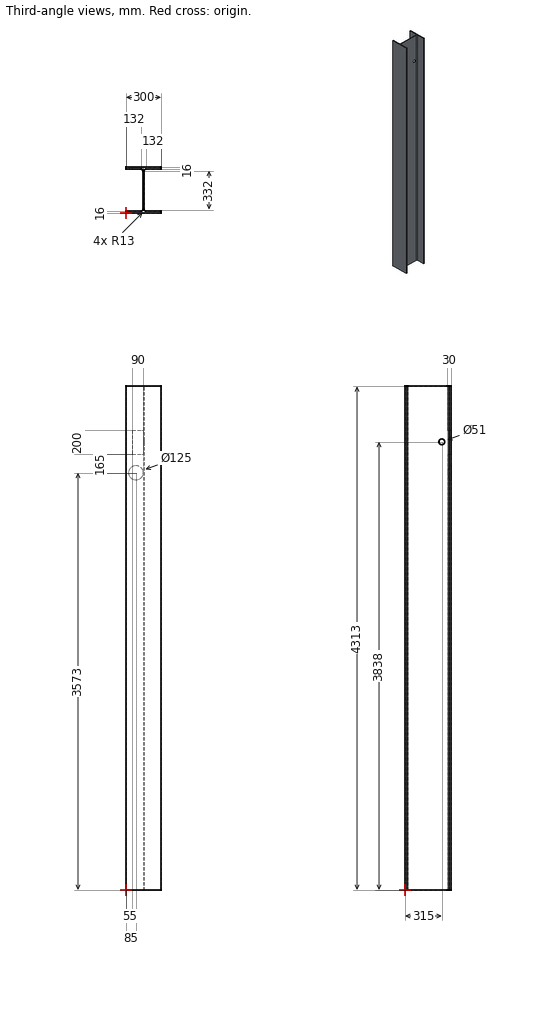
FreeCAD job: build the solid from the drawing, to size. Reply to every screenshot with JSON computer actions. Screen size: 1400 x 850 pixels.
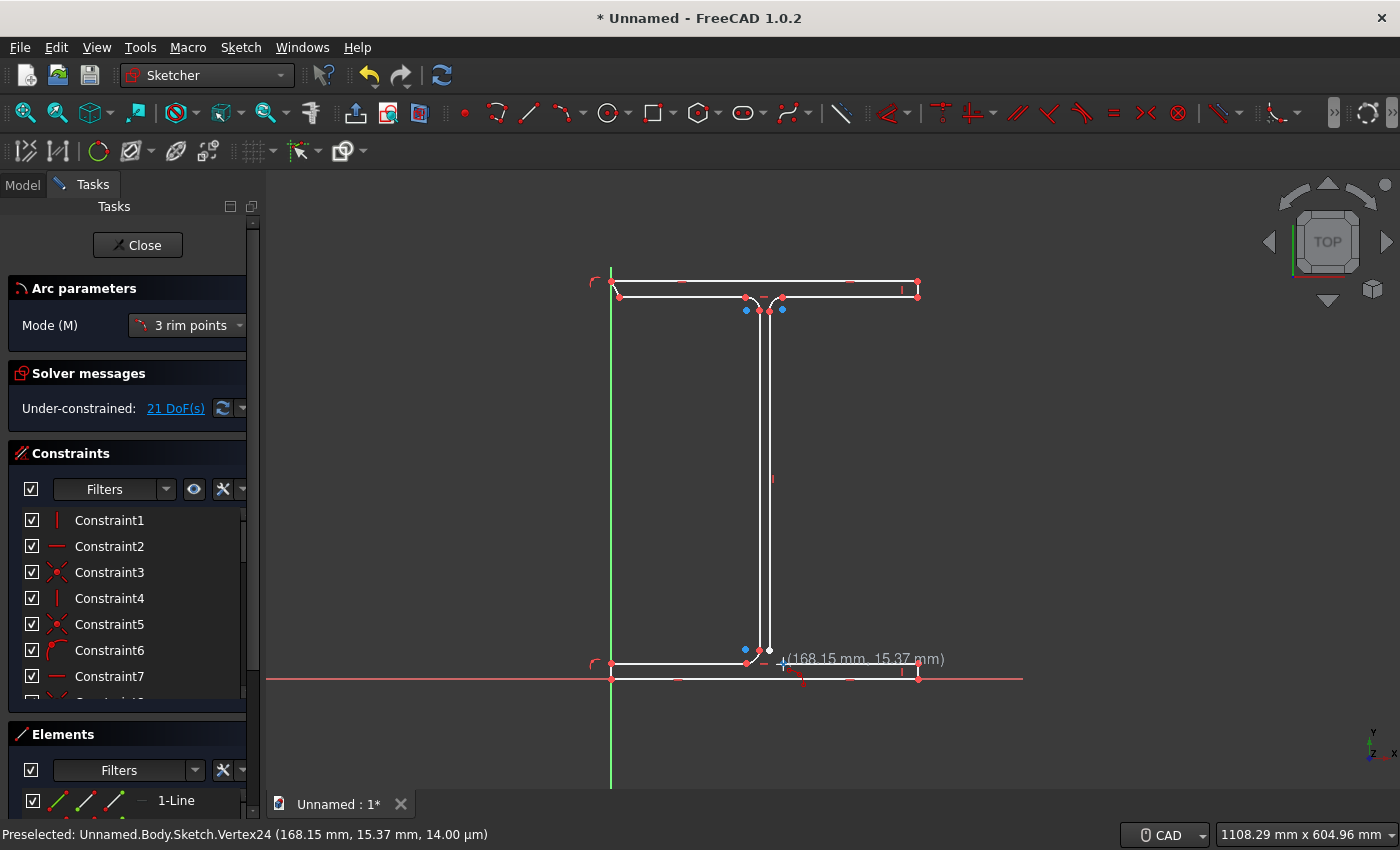
{"action": "scroll", "coordinate": [770, 650], "scroll_direction": "up", "scroll_amount": 3}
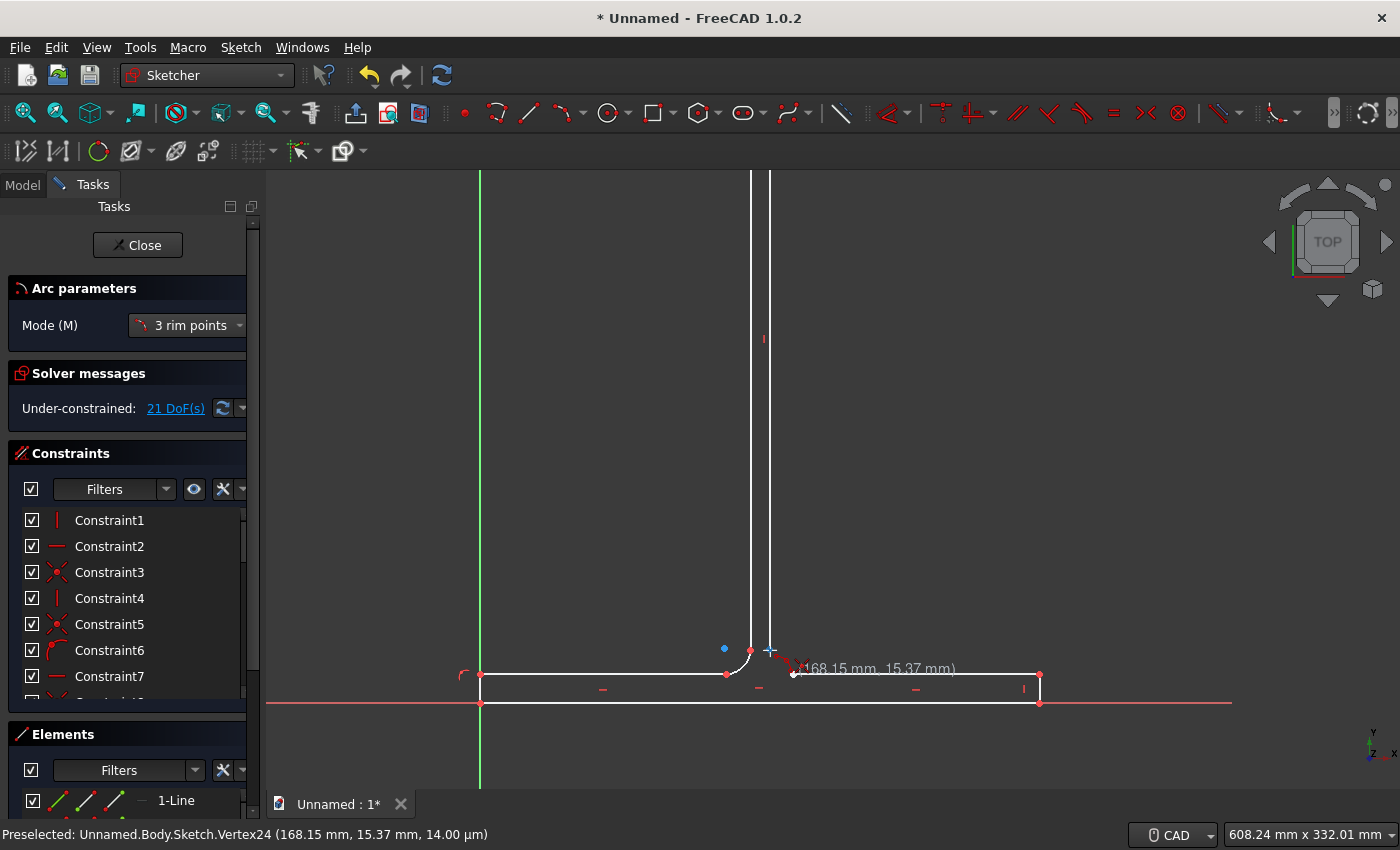
{"action": "left_click", "coordinate": [770, 650]}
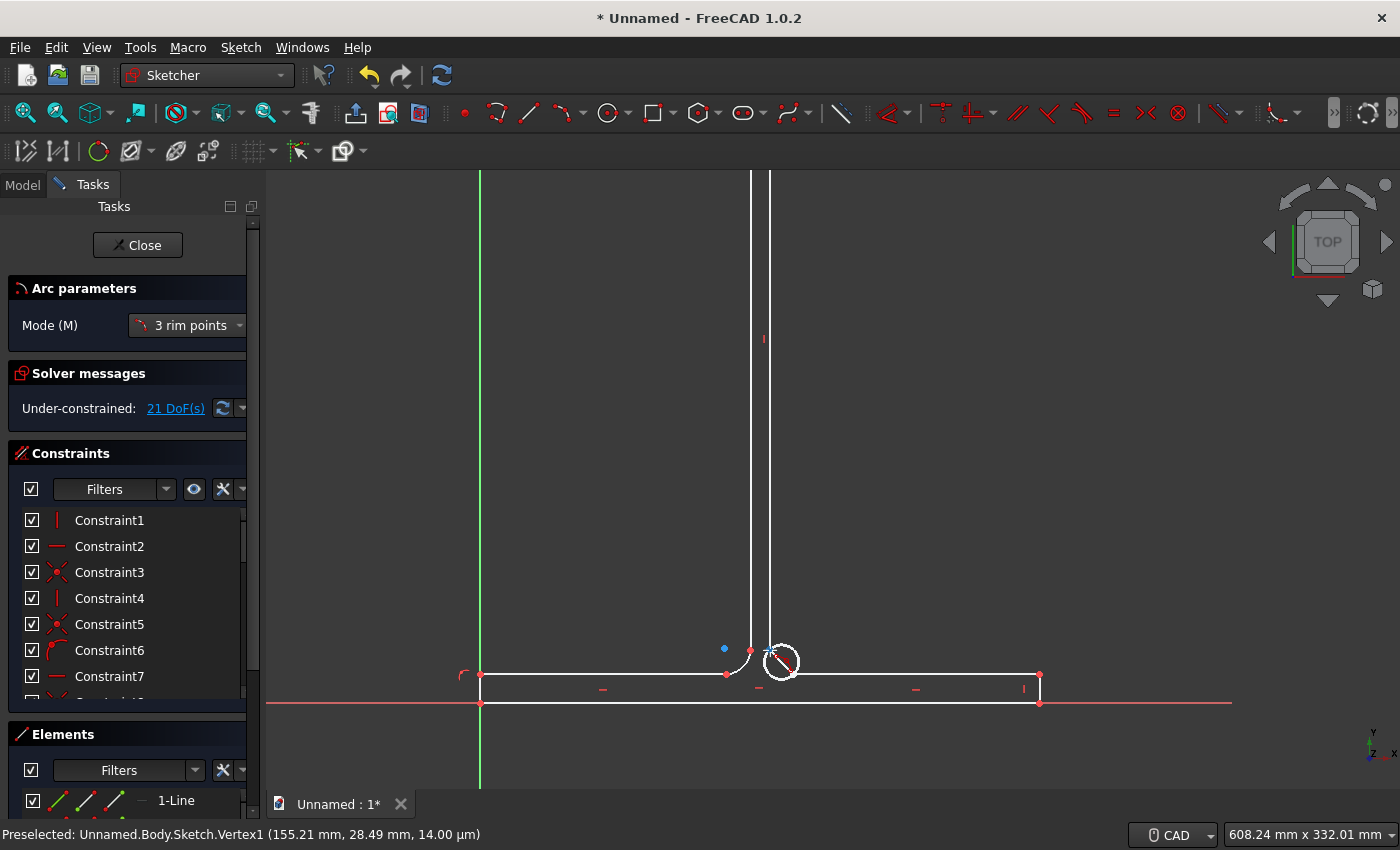
{"action": "scroll", "coordinate": [776, 666], "scroll_direction": "up", "scroll_amount": 5}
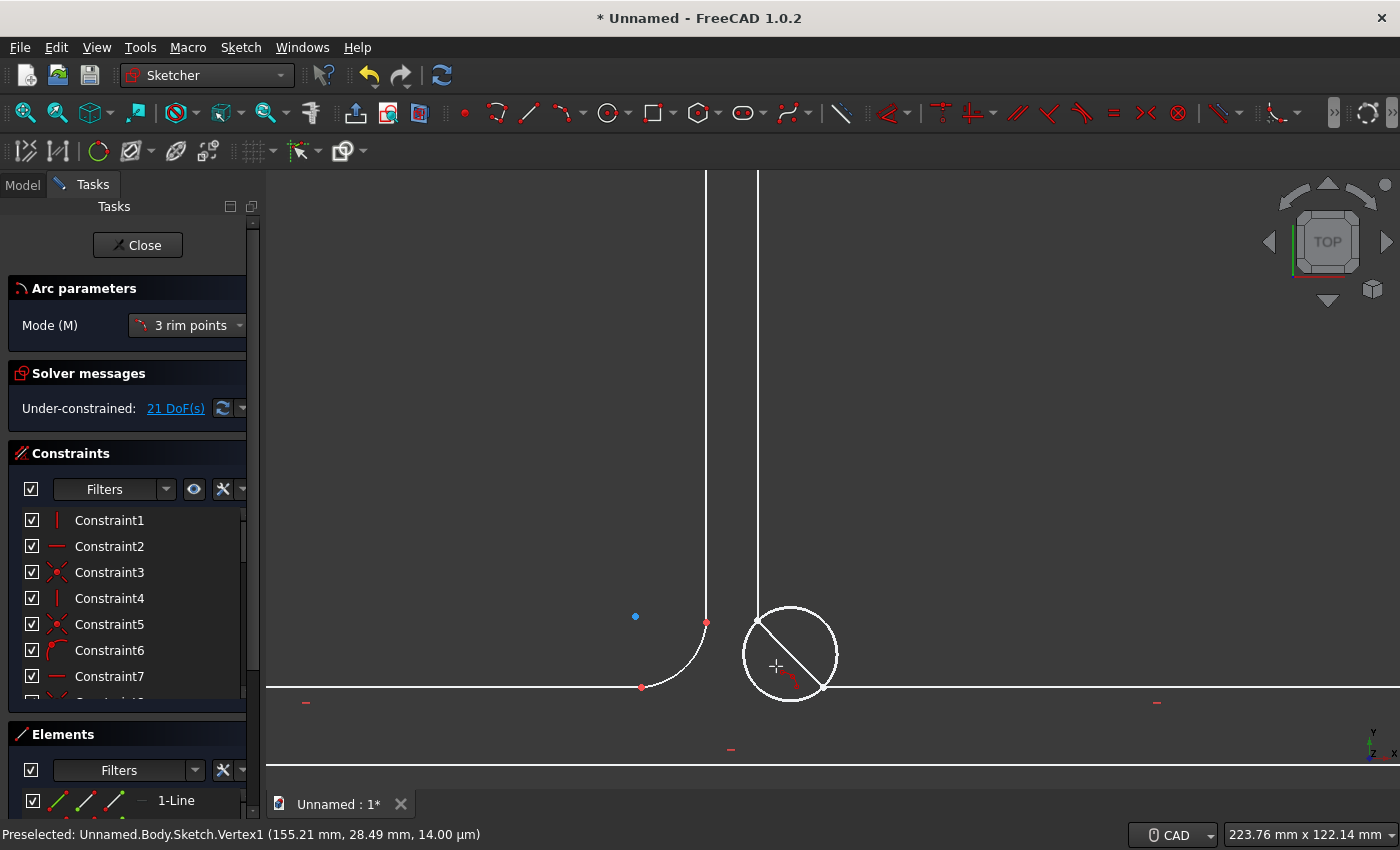
{"action": "left_click", "coordinate": [776, 665]}
{"action": "key", "text": "Escape"}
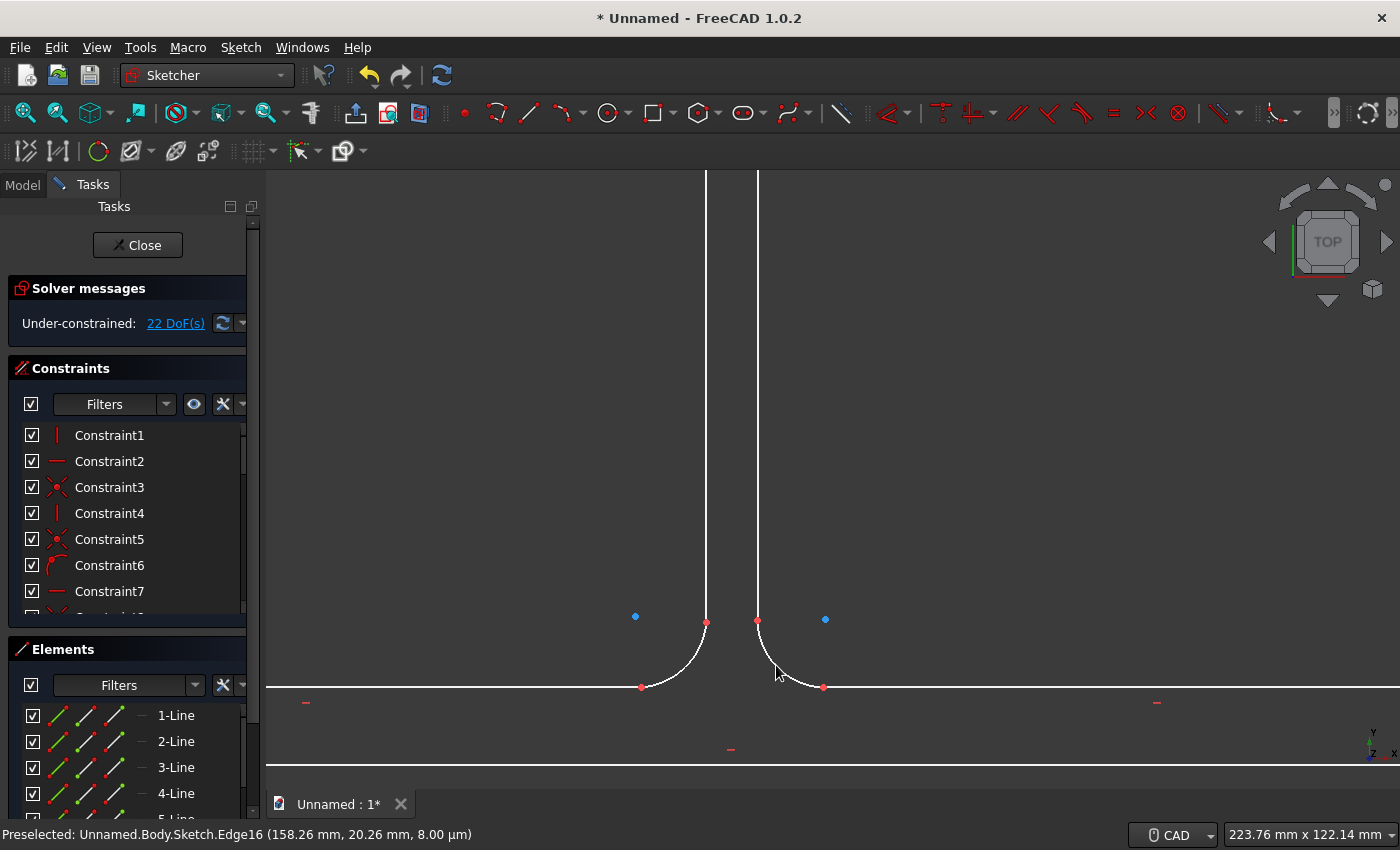
{"action": "scroll", "coordinate": [773, 657], "scroll_direction": "down", "scroll_amount": 8}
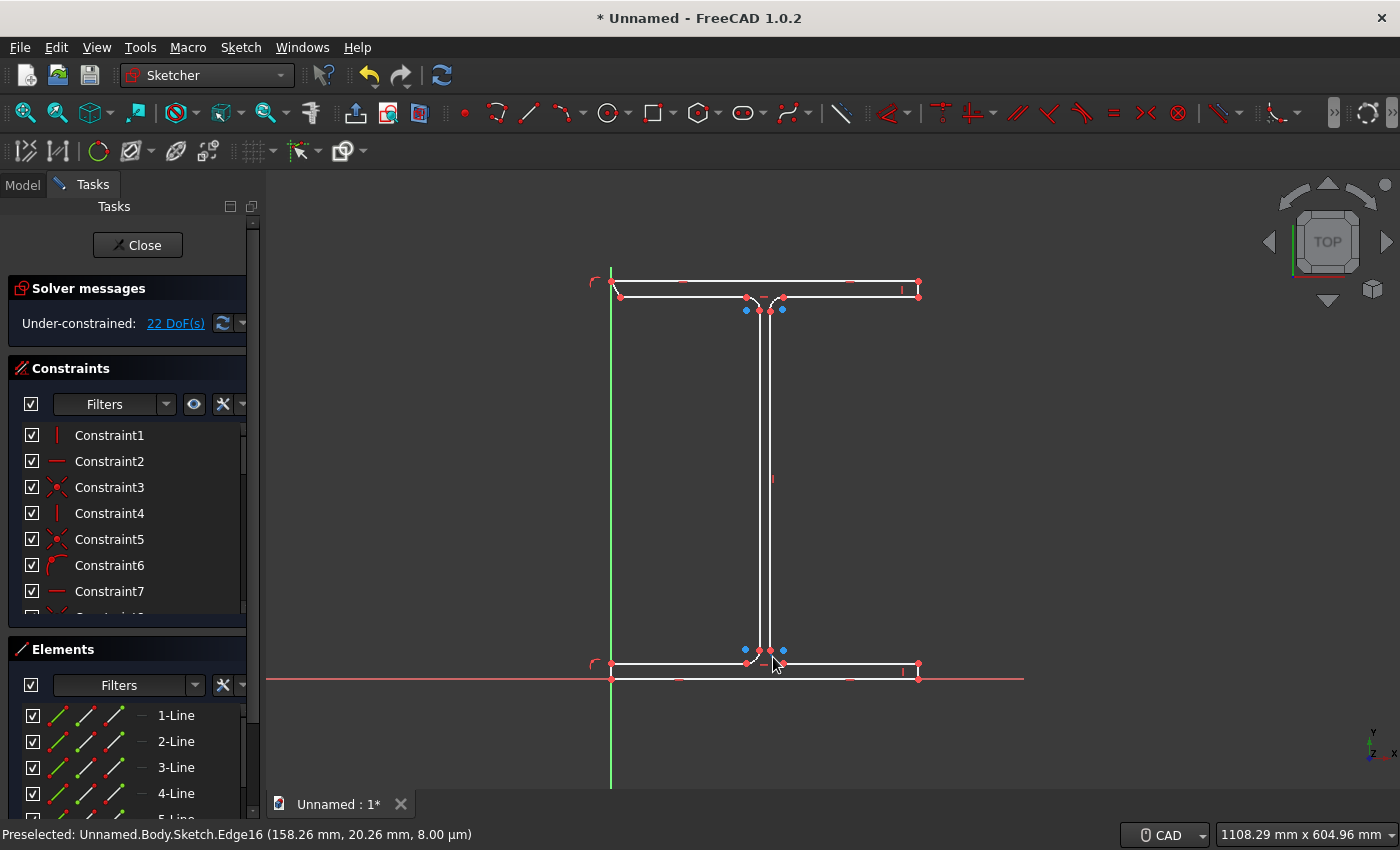
{"action": "scroll", "coordinate": [770, 583], "scroll_direction": "up", "scroll_amount": 2}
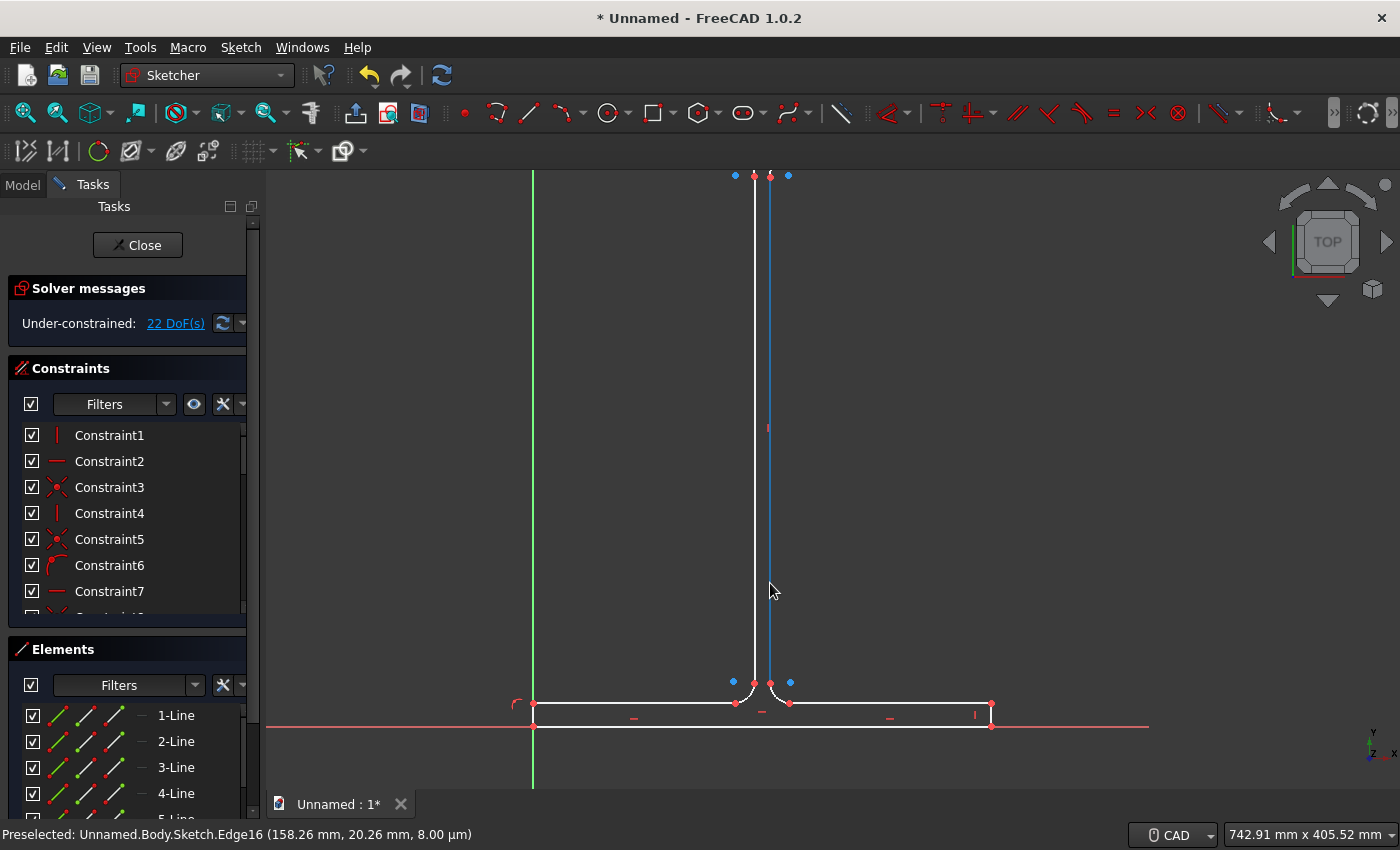
{"action": "left_click", "coordinate": [770, 582]}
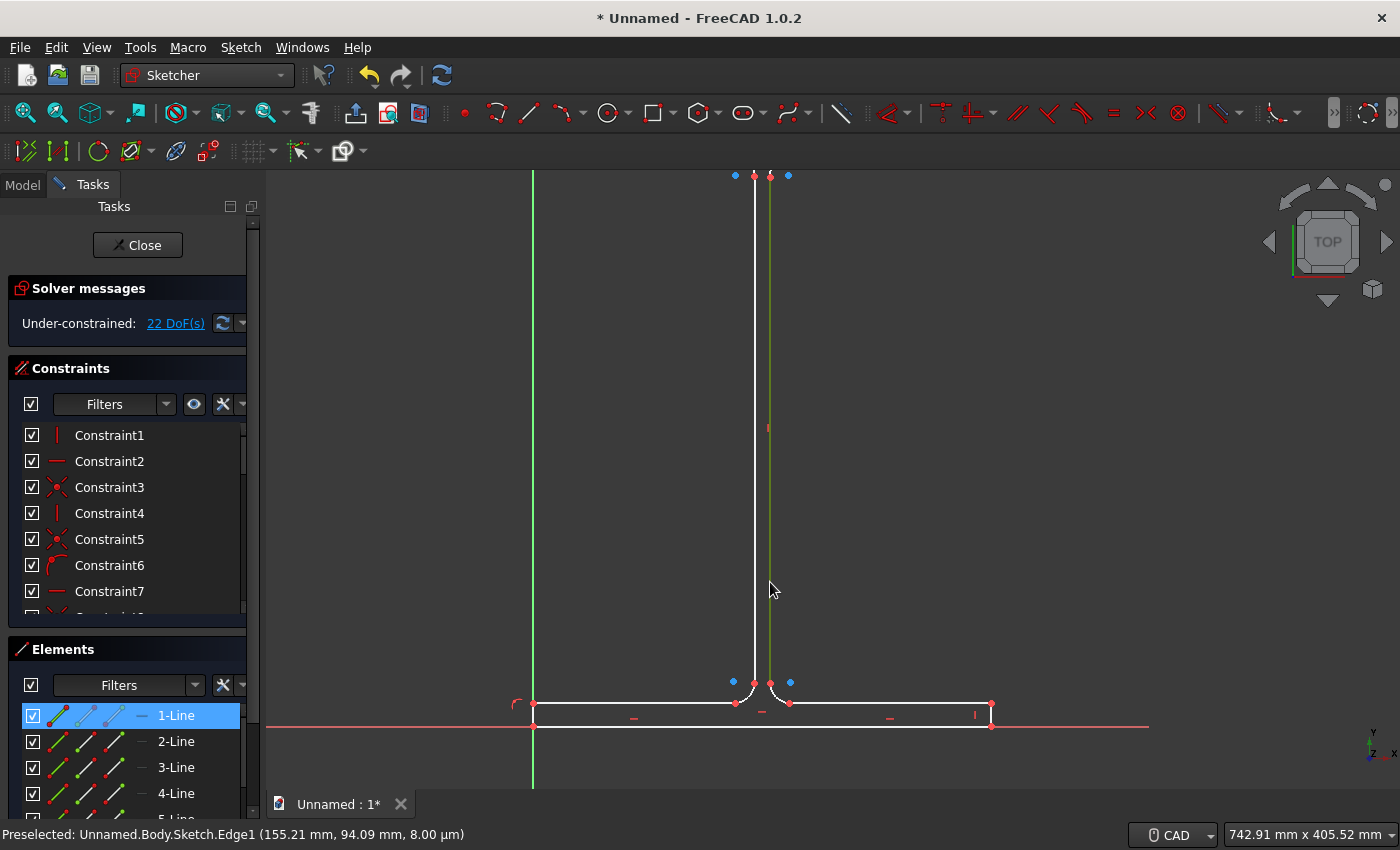
{"action": "scroll", "coordinate": [769, 582], "scroll_direction": "down", "scroll_amount": 2}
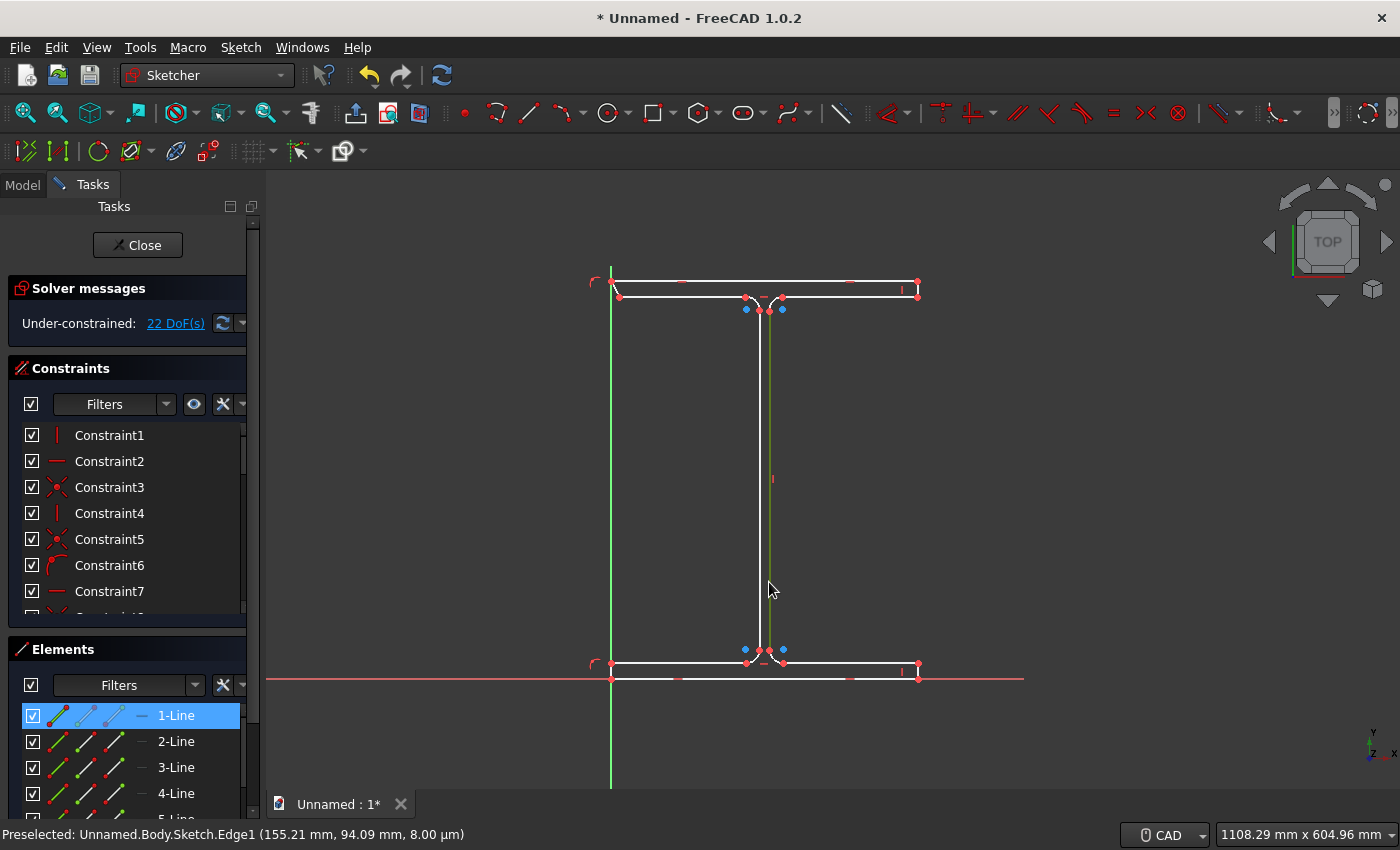
{"action": "scroll", "coordinate": [777, 298], "scroll_direction": "up", "scroll_amount": 4}